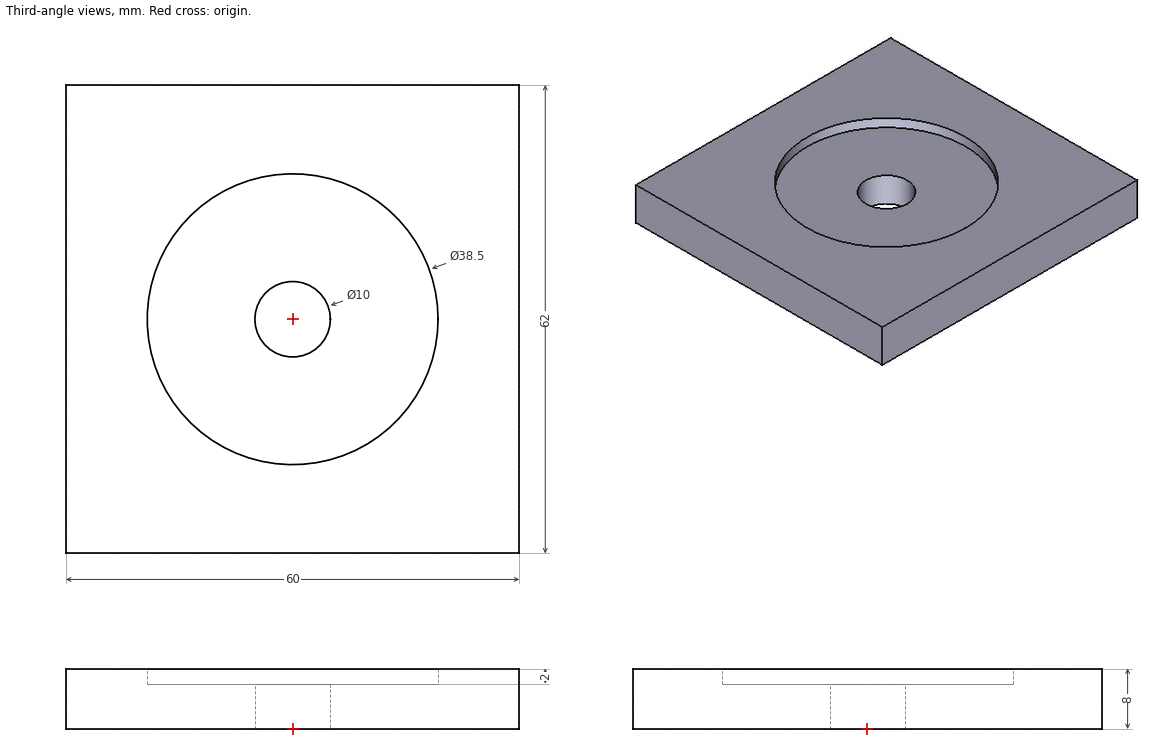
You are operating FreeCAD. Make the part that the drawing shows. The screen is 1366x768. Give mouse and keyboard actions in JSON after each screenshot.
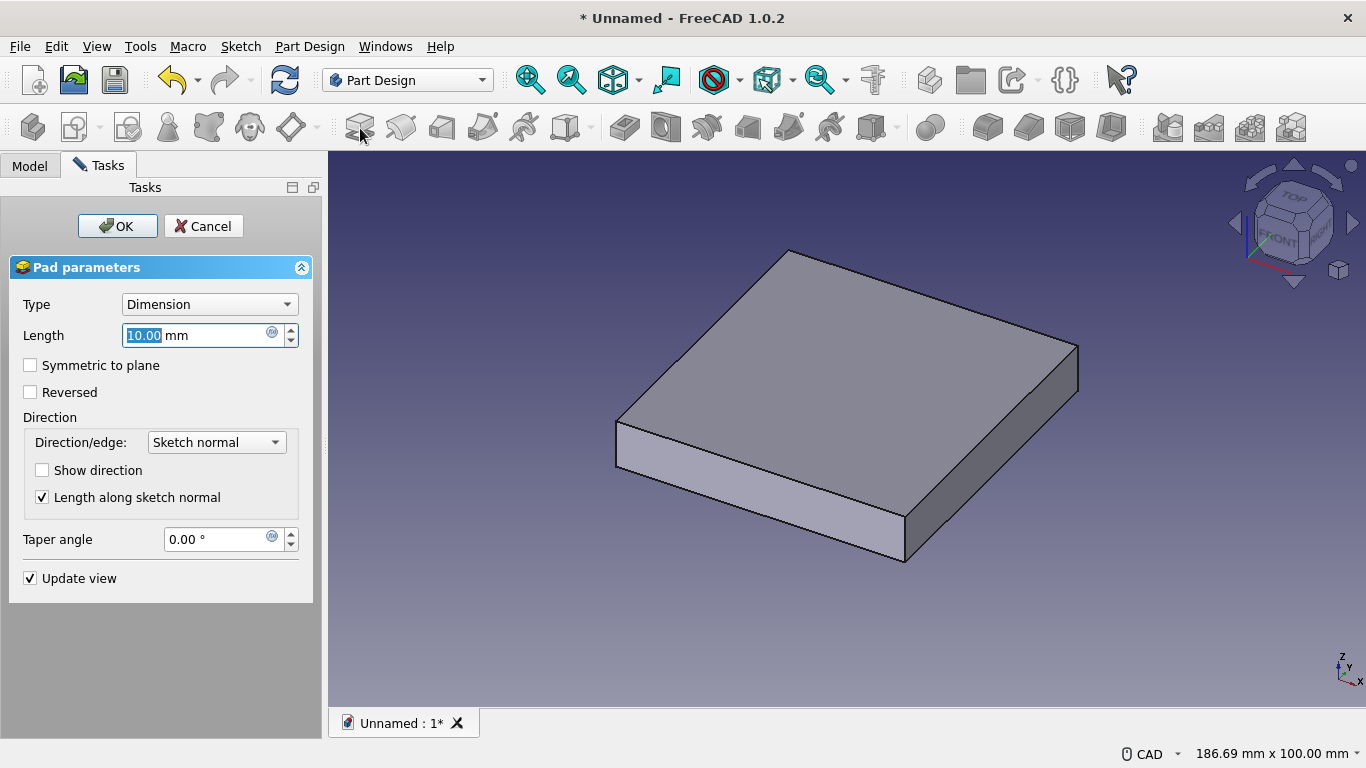
{"action": "type", "text": "8"}
{"action": "key", "text": "Tab"}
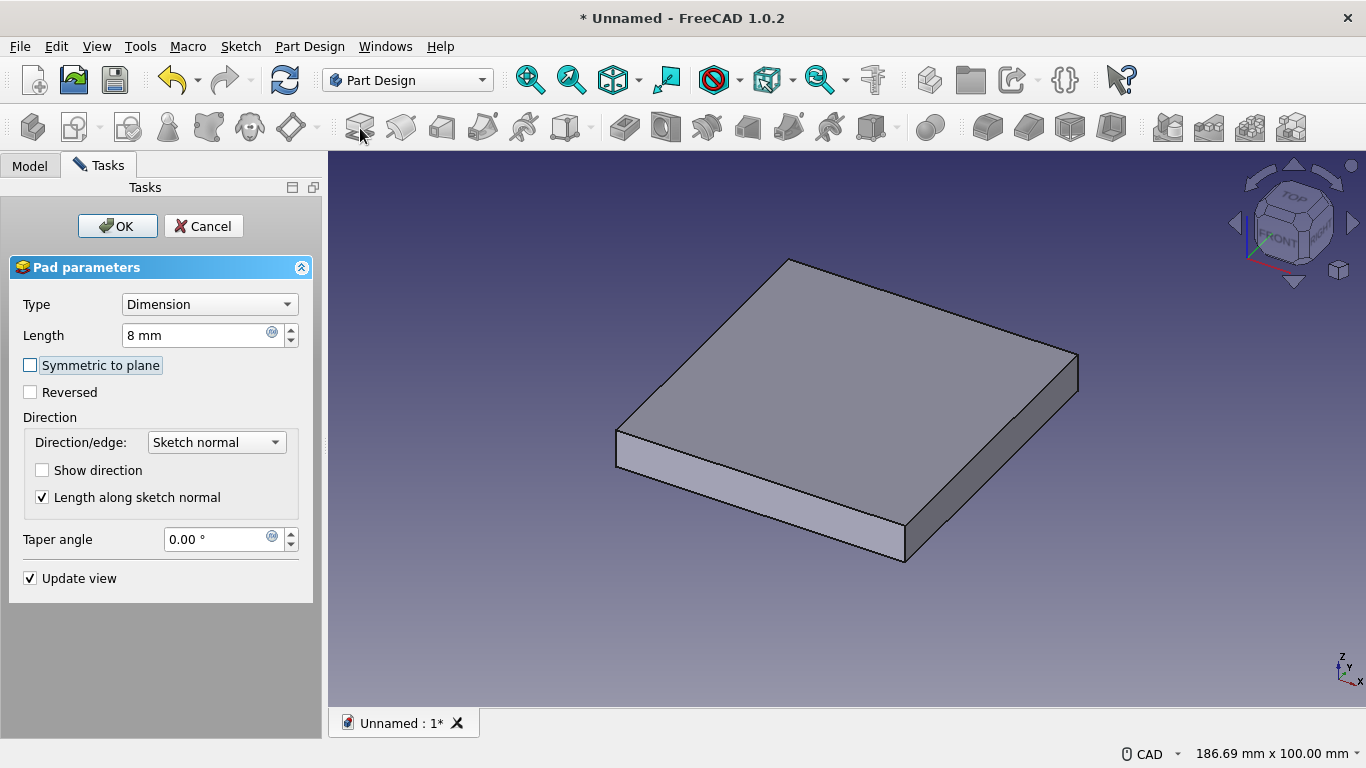
{"action": "left_click", "coordinate": [118, 226]}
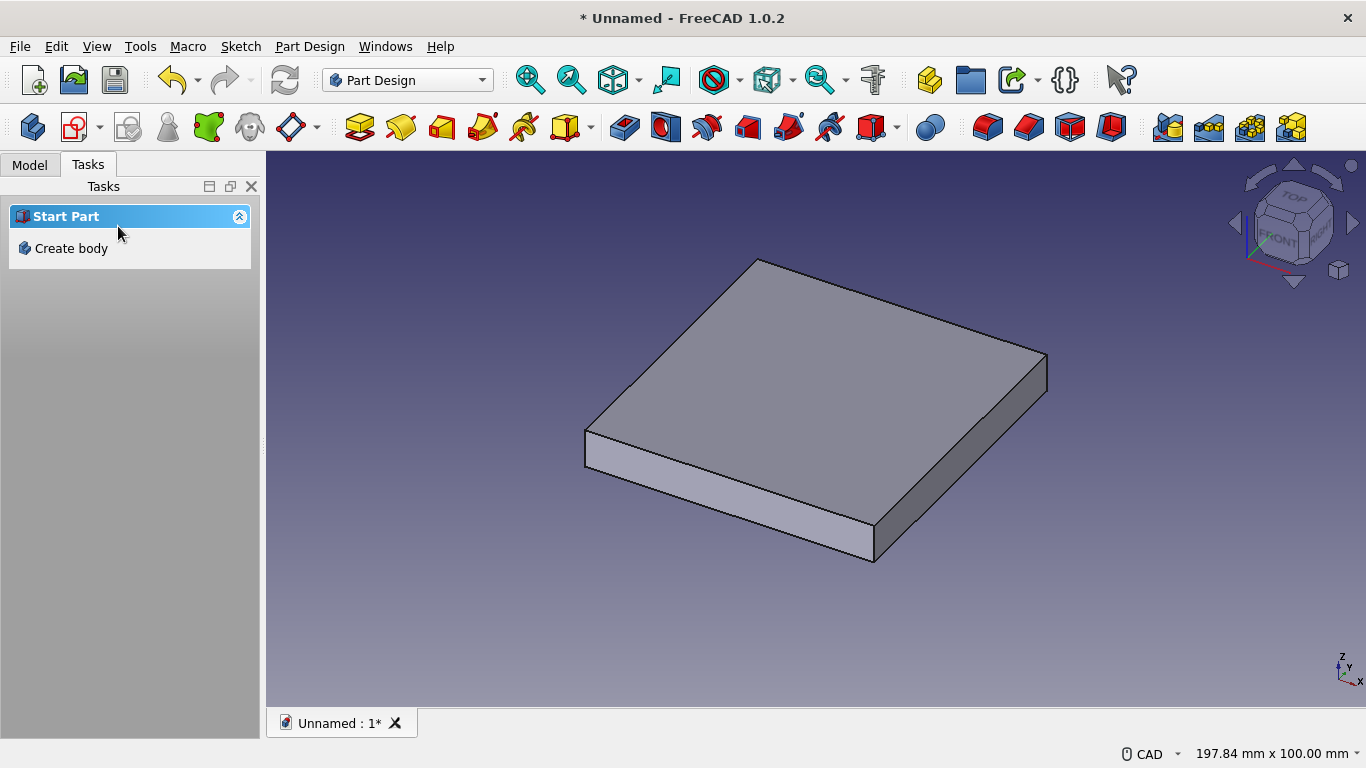
{"action": "left_click", "coordinate": [816, 392]}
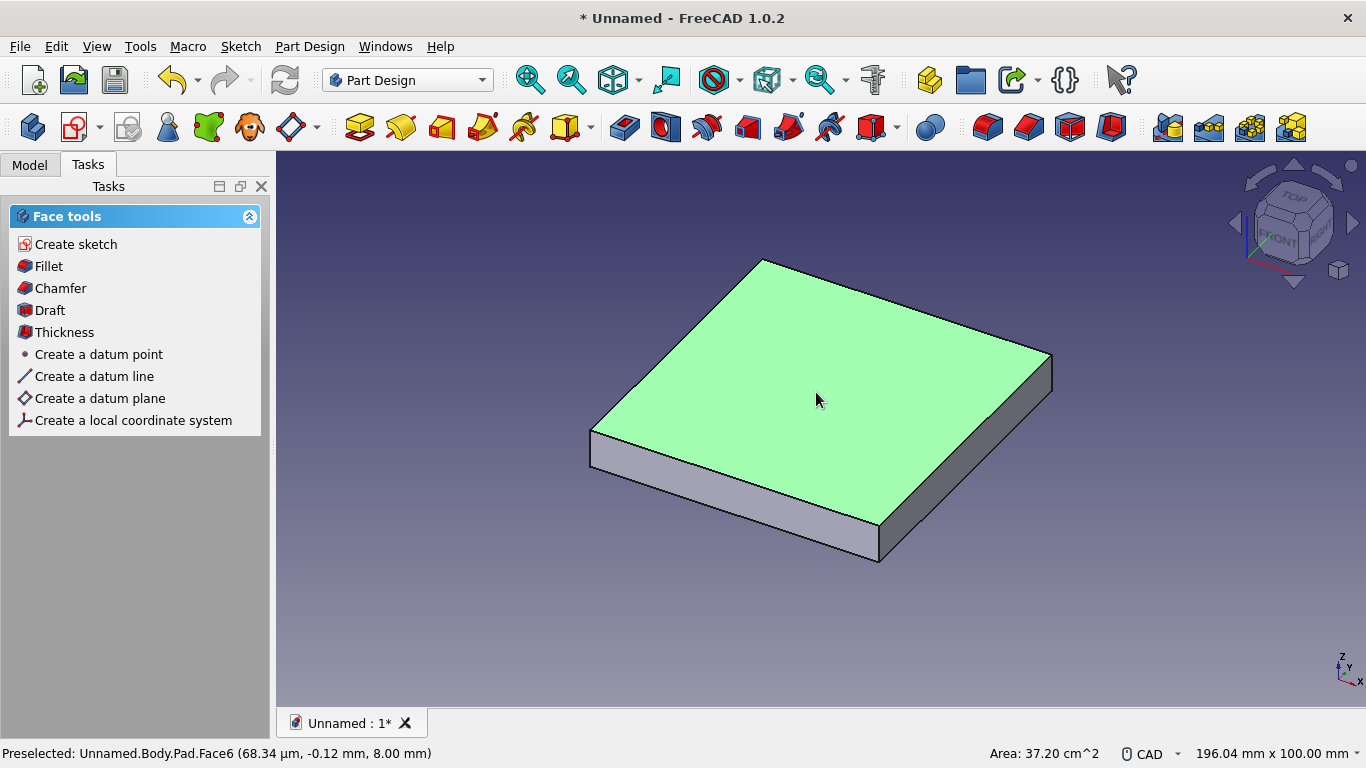
{"action": "left_click", "coordinate": [74, 128]}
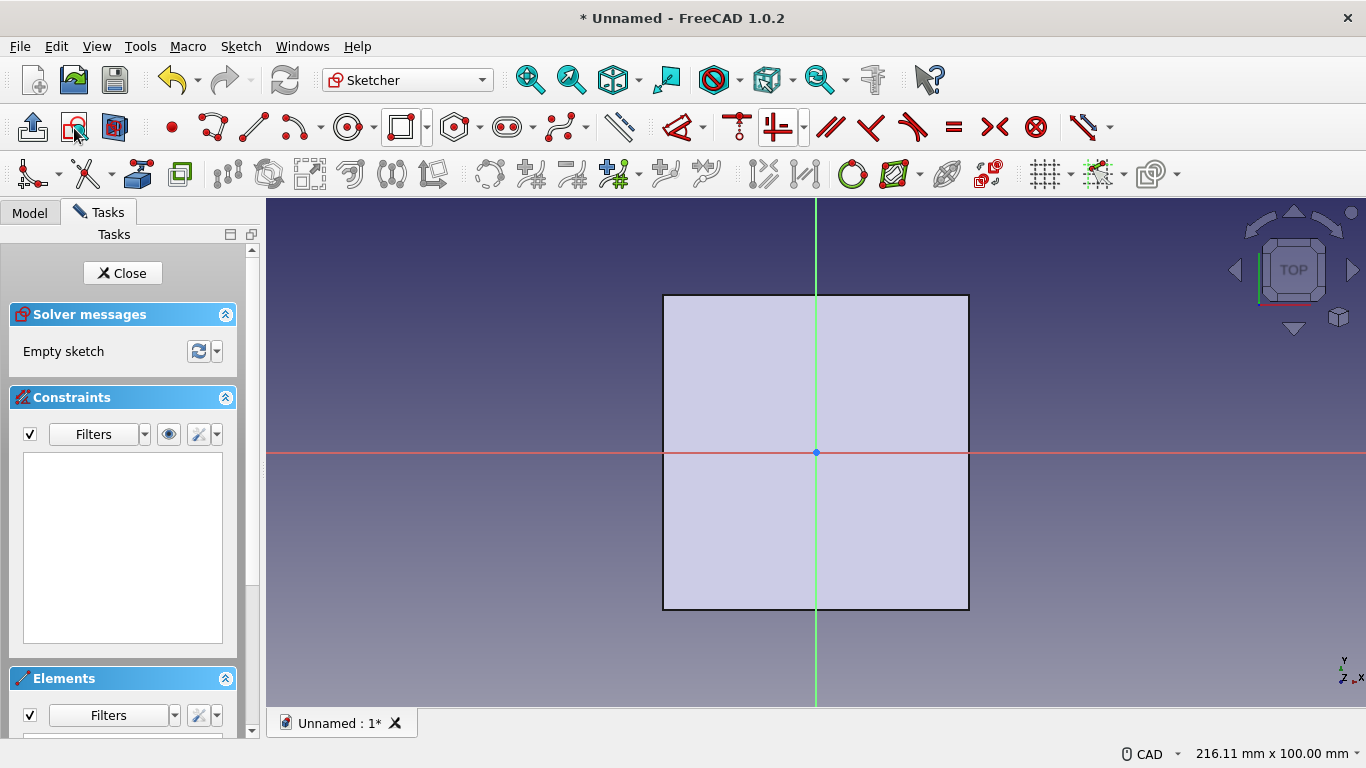
{"action": "scroll", "coordinate": [955, 453], "scroll_direction": "up", "scroll_amount": 2}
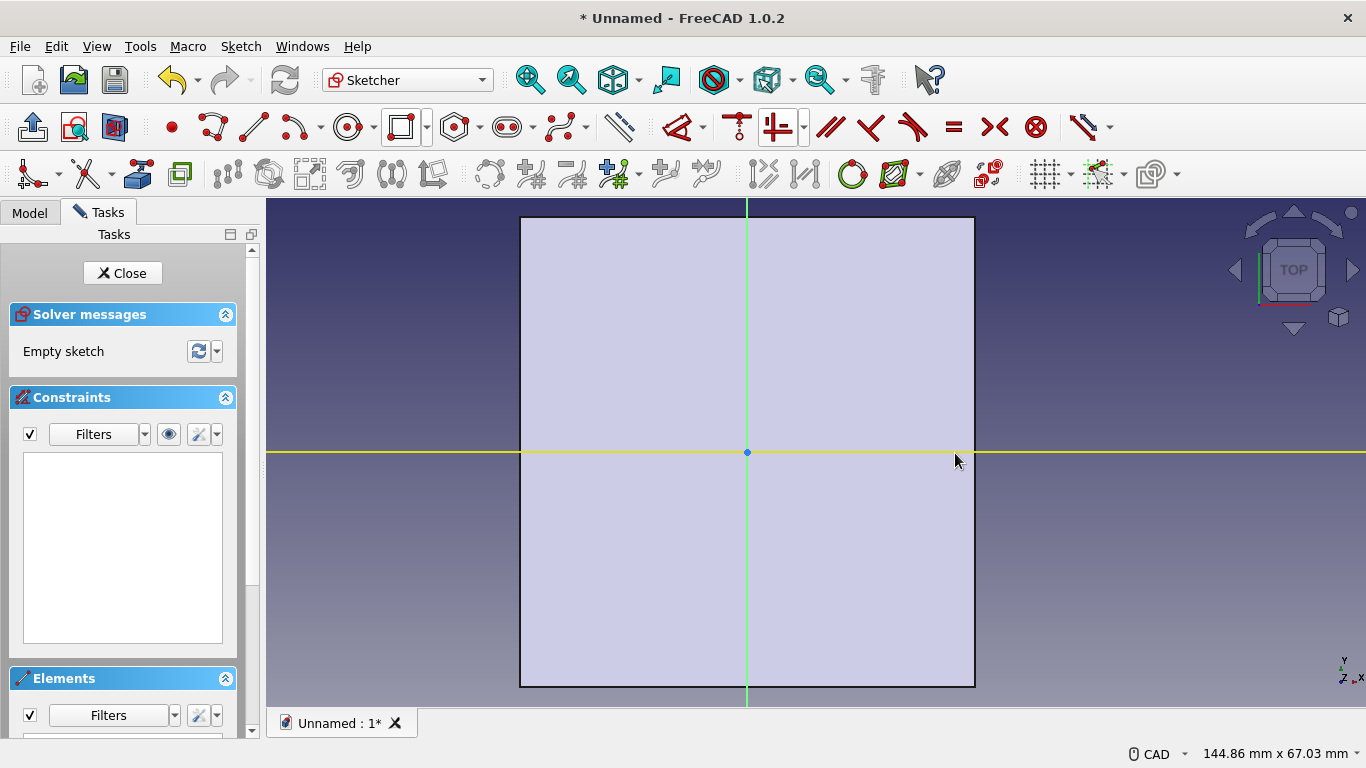
{"action": "key", "text": "g c"}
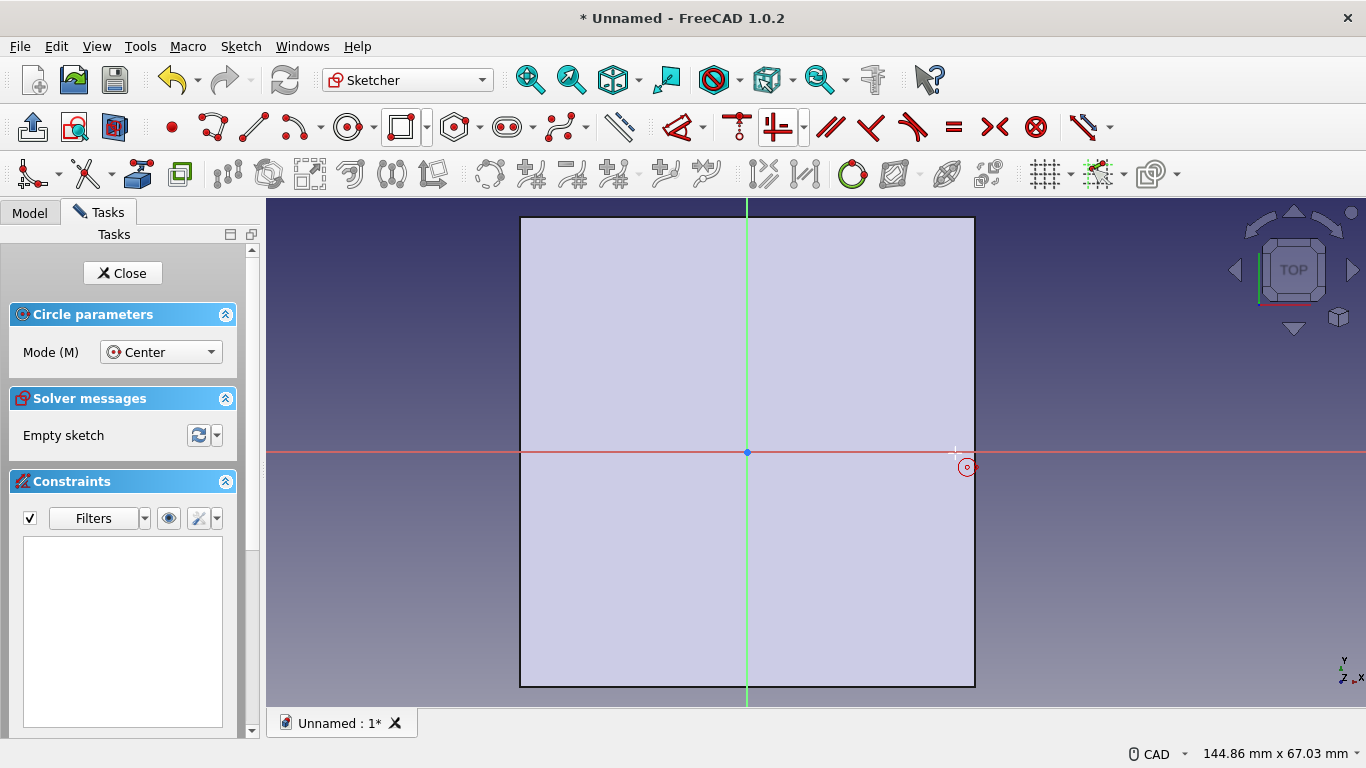
{"action": "left_click", "coordinate": [747, 452]}
{"action": "mouse_move", "coordinate": [851, 349]}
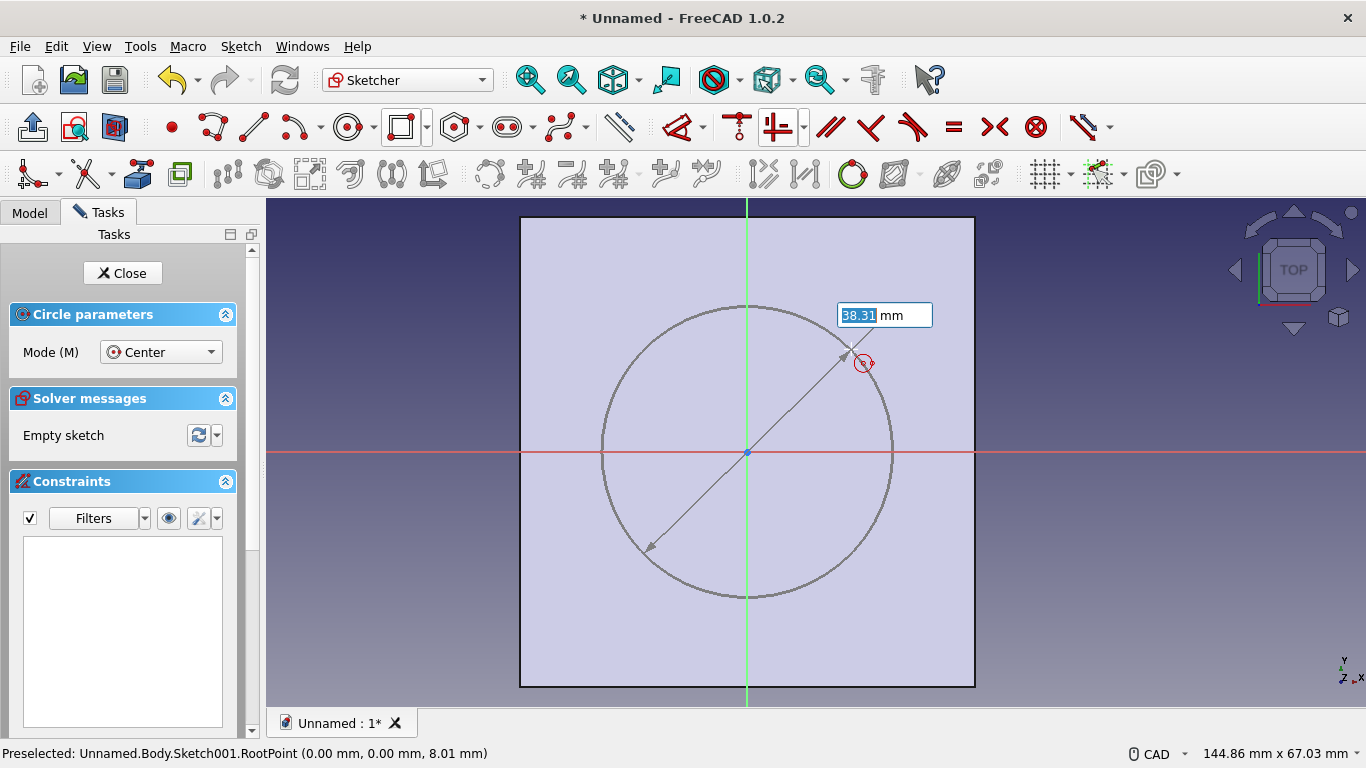
{"action": "type", "text": "38.5"}
{"action": "key", "text": "Return"}
{"action": "key", "text": "Escape"}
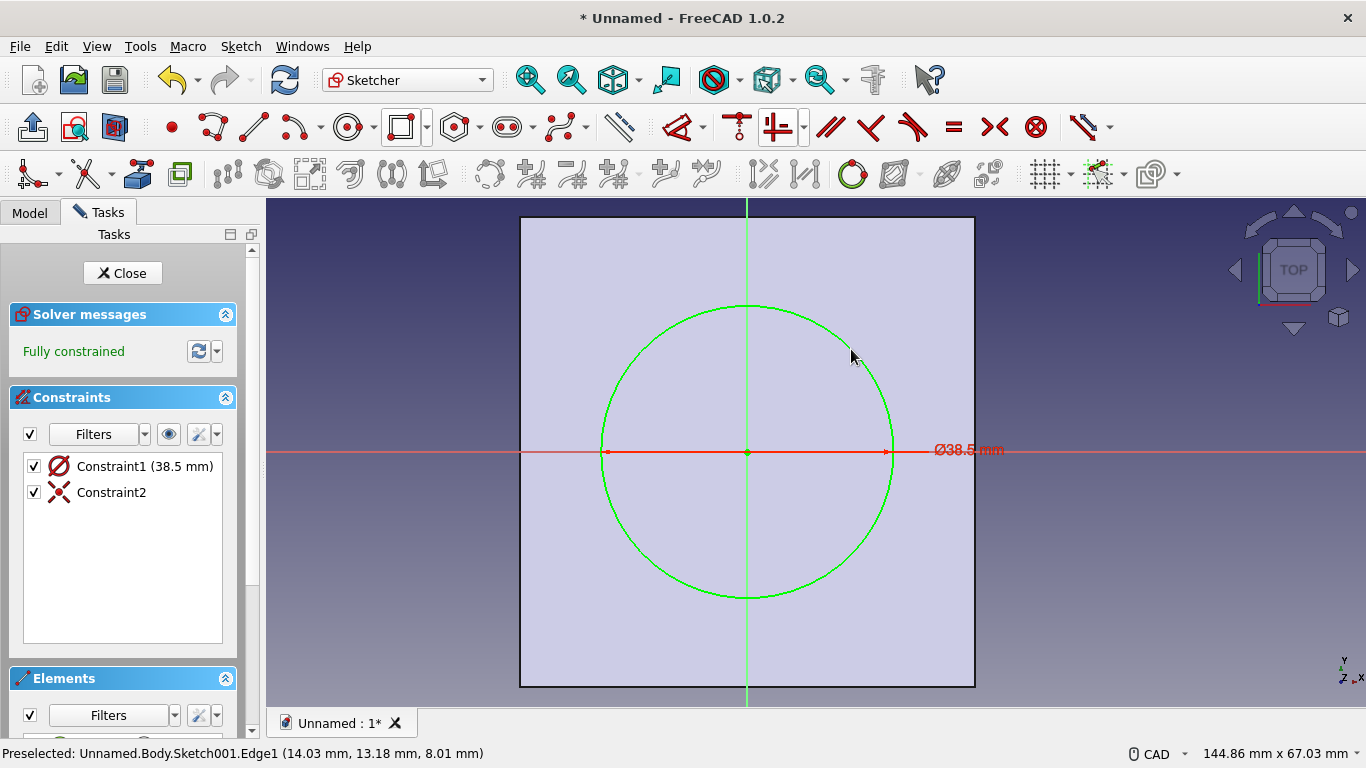
{"action": "left_click", "coordinate": [123, 273]}